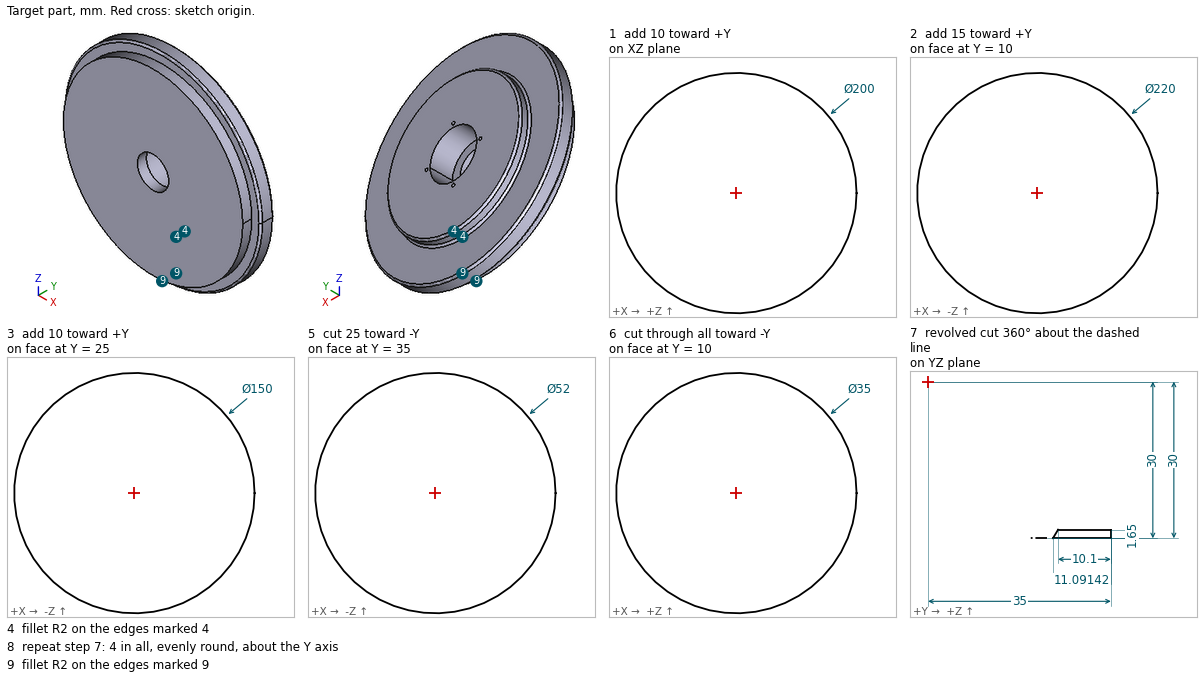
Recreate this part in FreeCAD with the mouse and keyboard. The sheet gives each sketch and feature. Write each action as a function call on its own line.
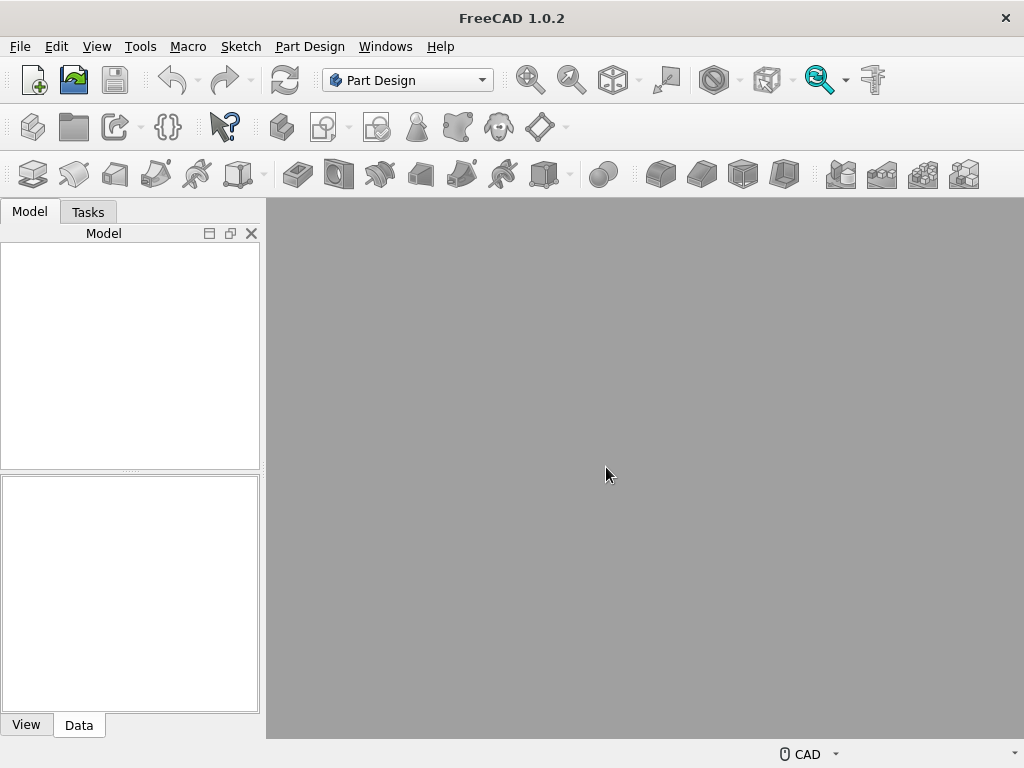
click(33, 80)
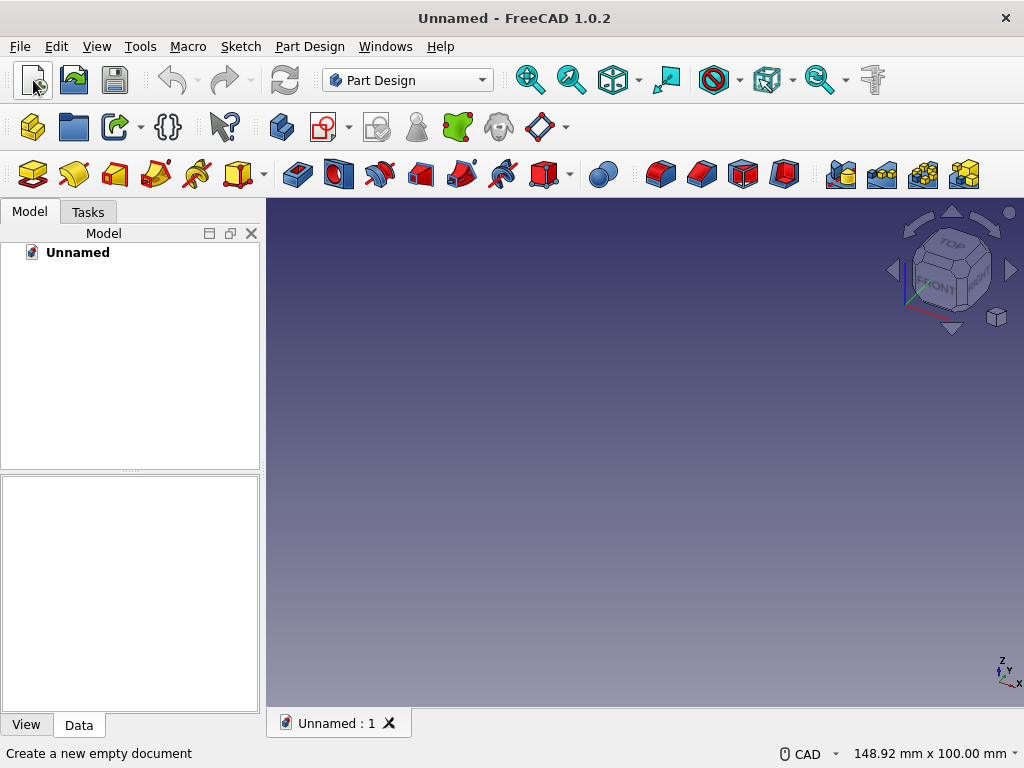
click(322, 128)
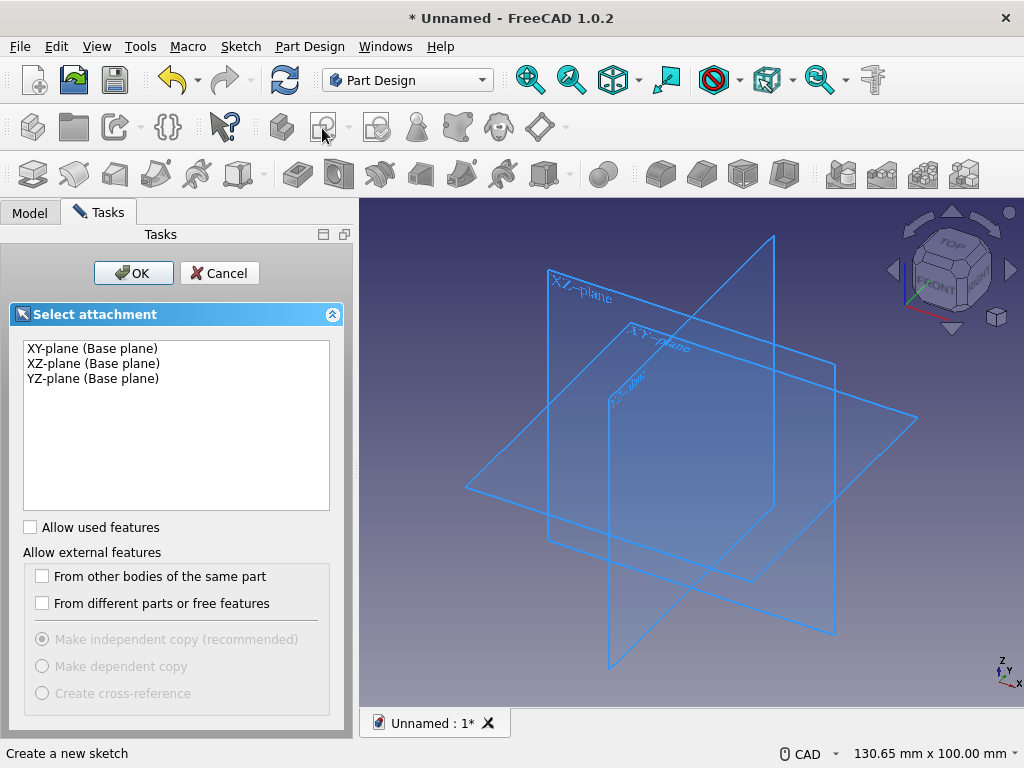
click(84, 364)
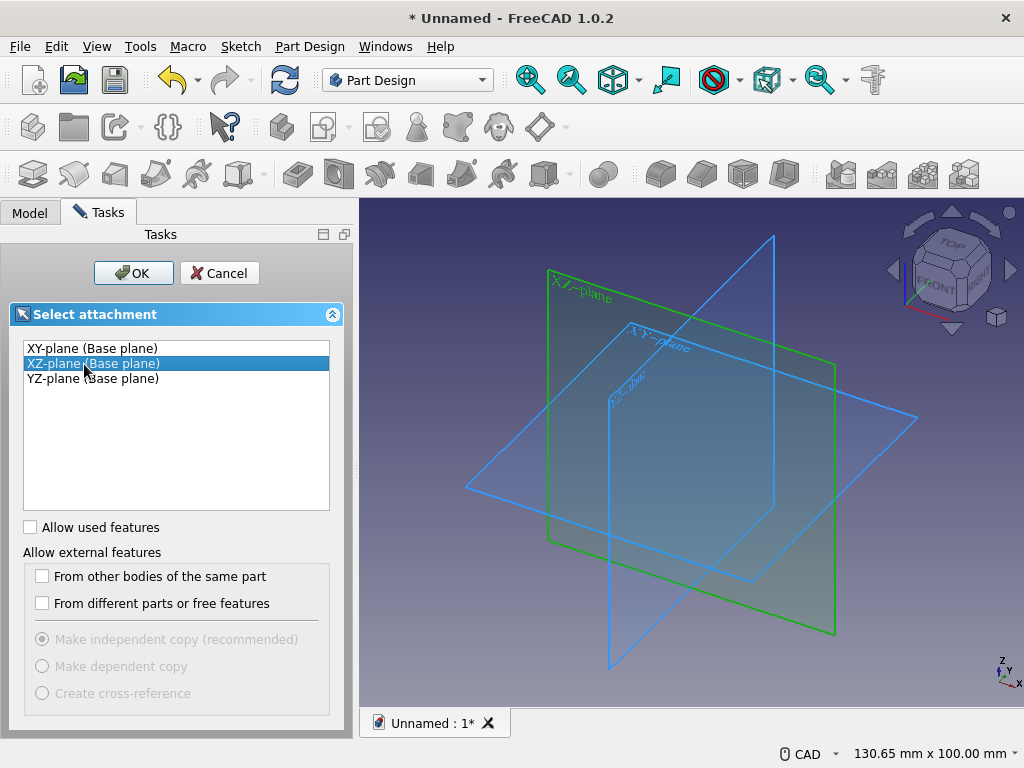
click(134, 273)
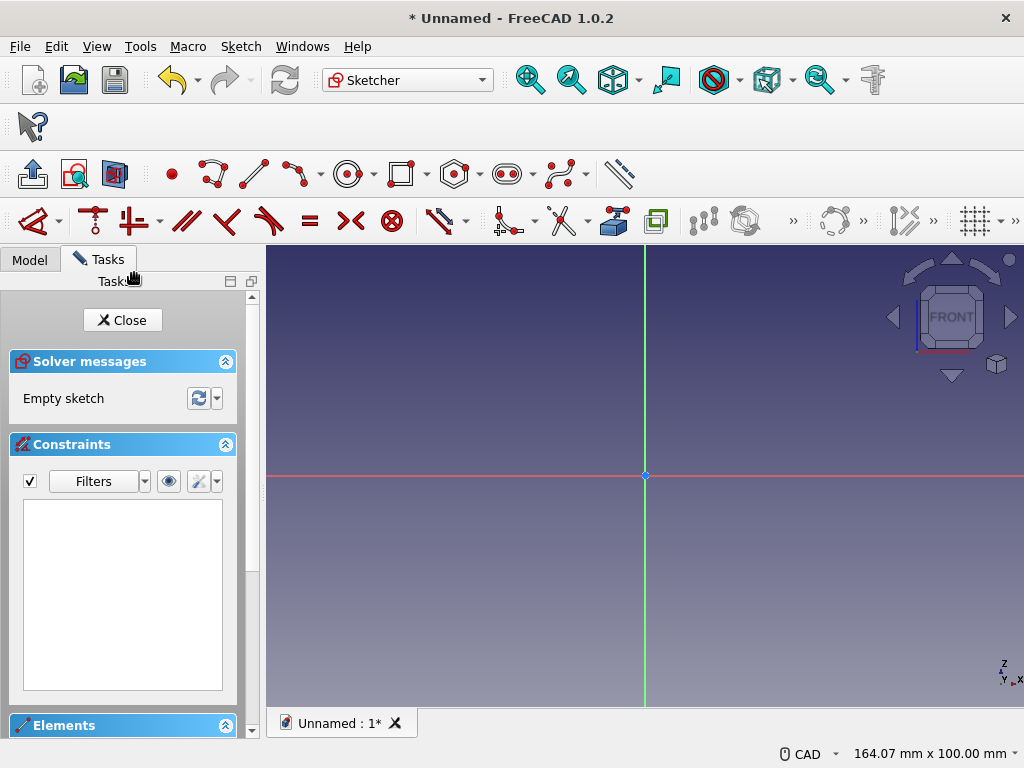
scroll(547, 476, down, 6)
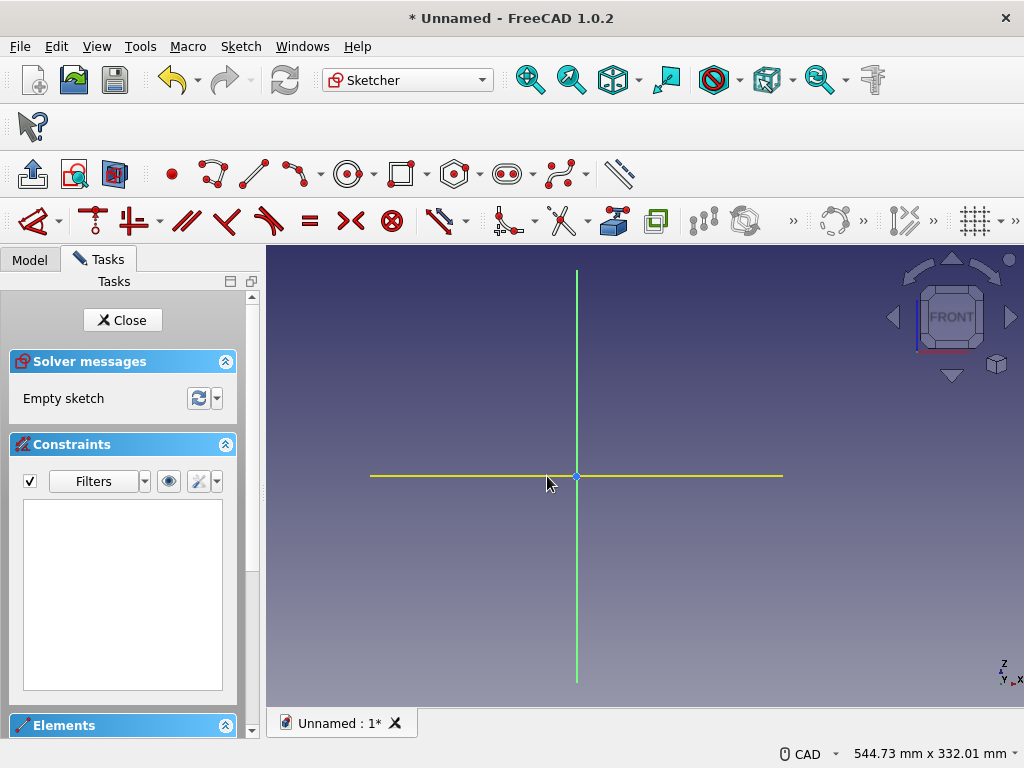
click(348, 174)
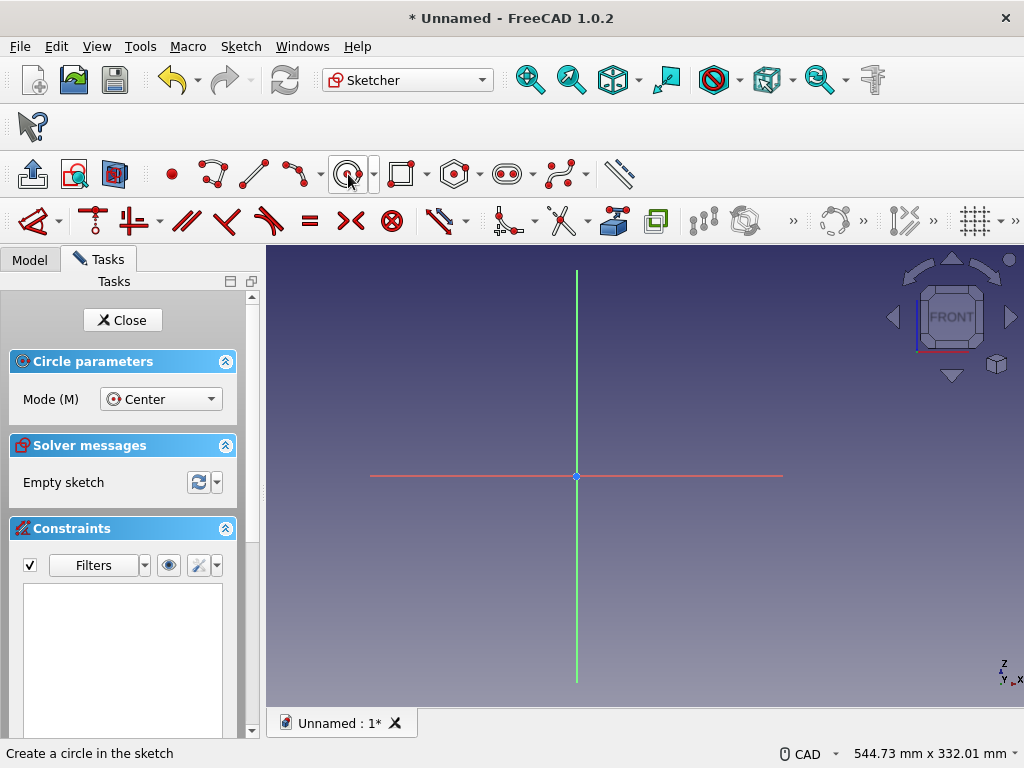
click(577, 476)
click(675, 378)
key(Escape)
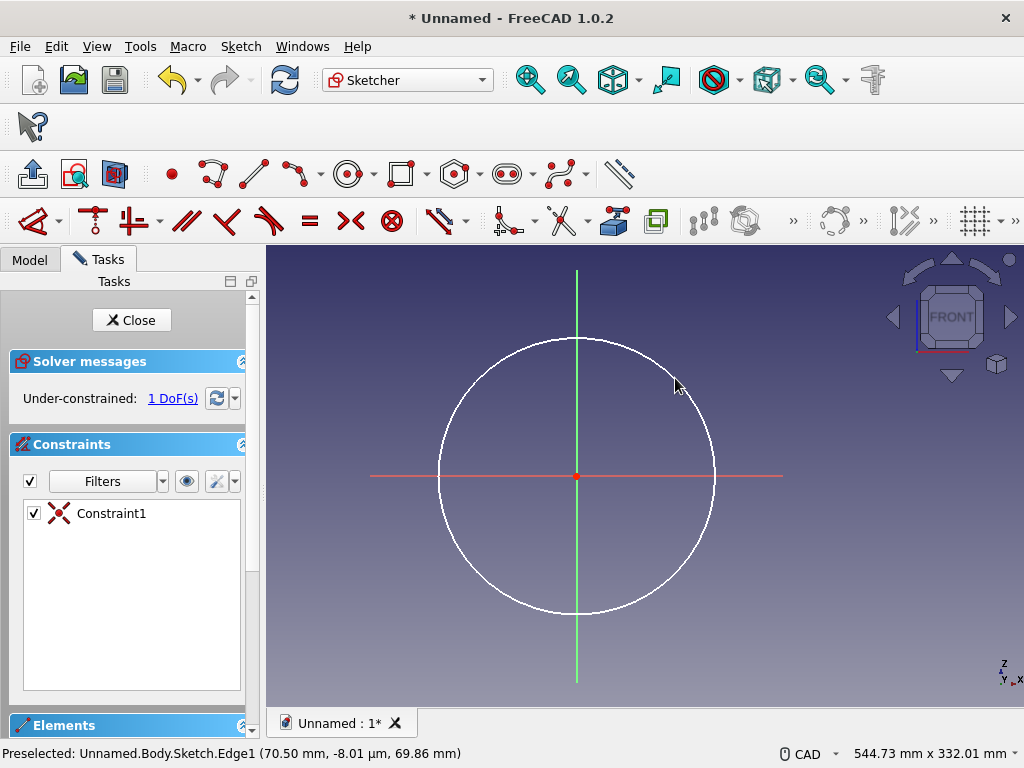
click(32, 222)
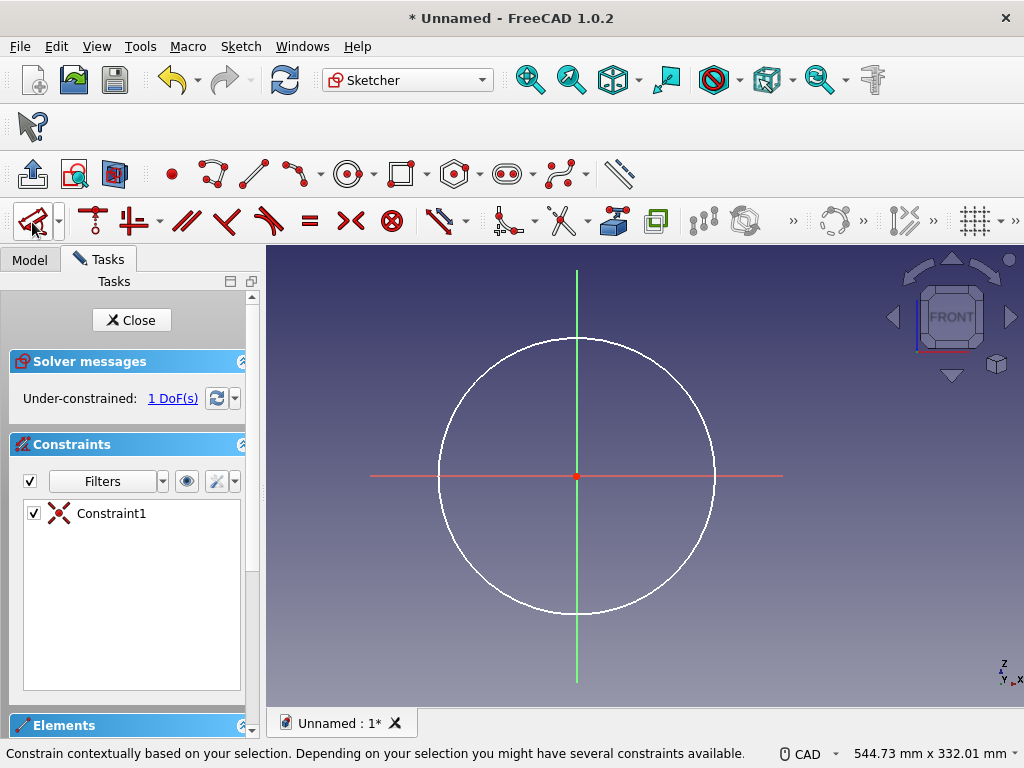
click(674, 378)
click(696, 355)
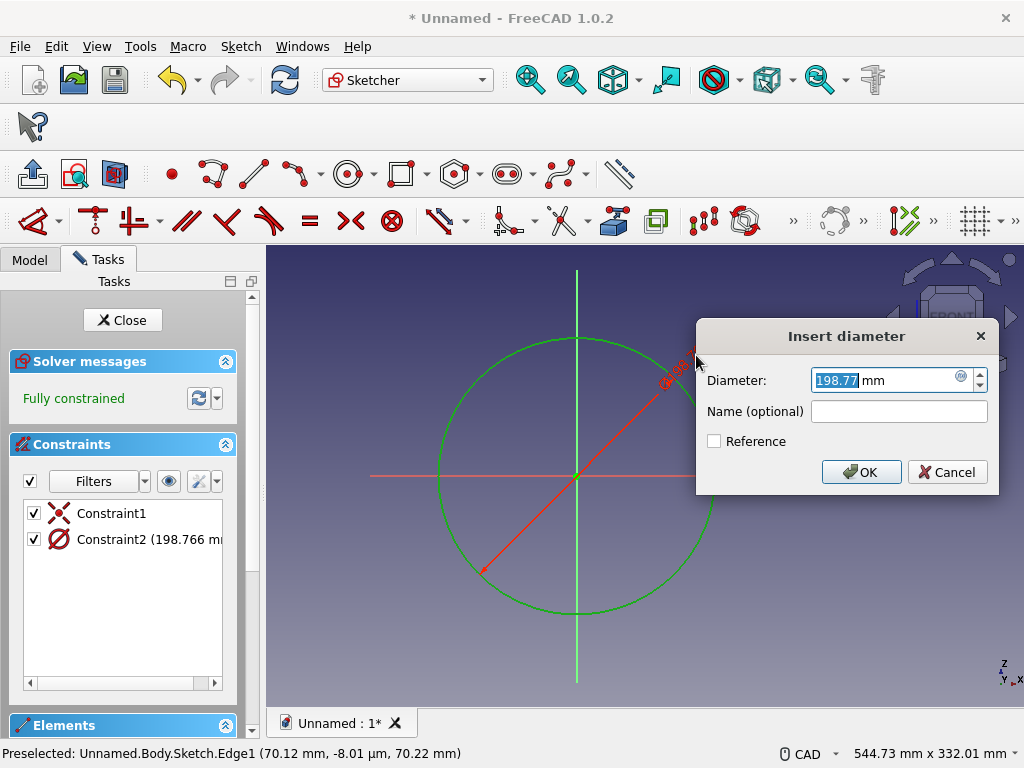
text(200)
key(Return)
key(Escape)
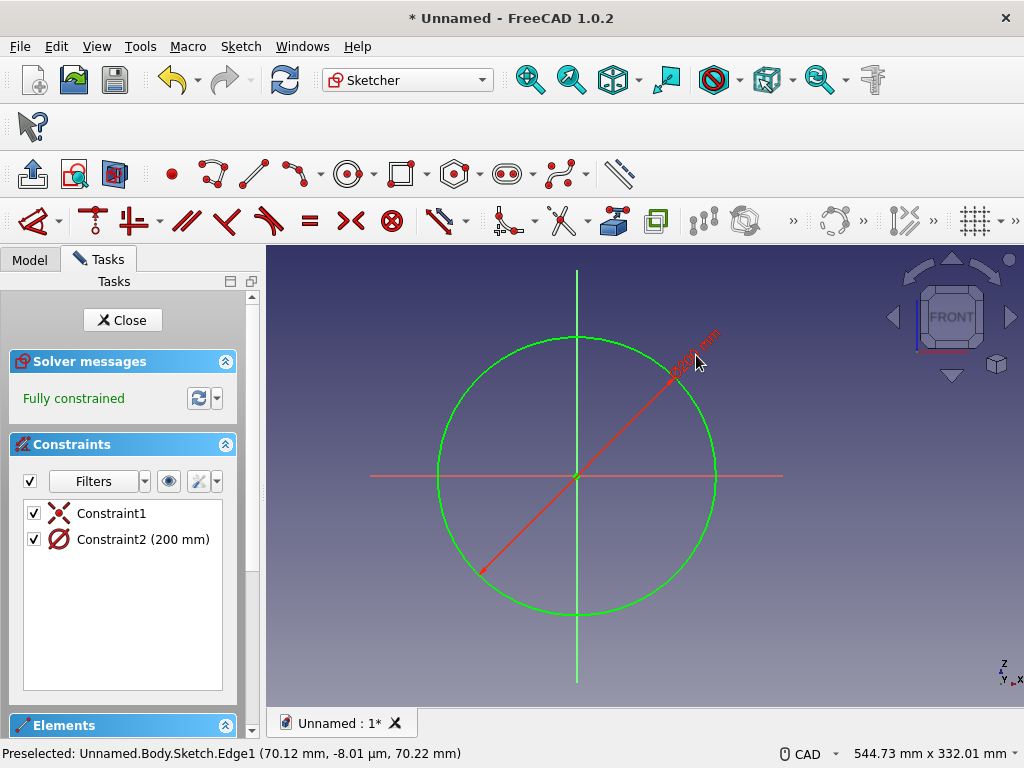
click(123, 320)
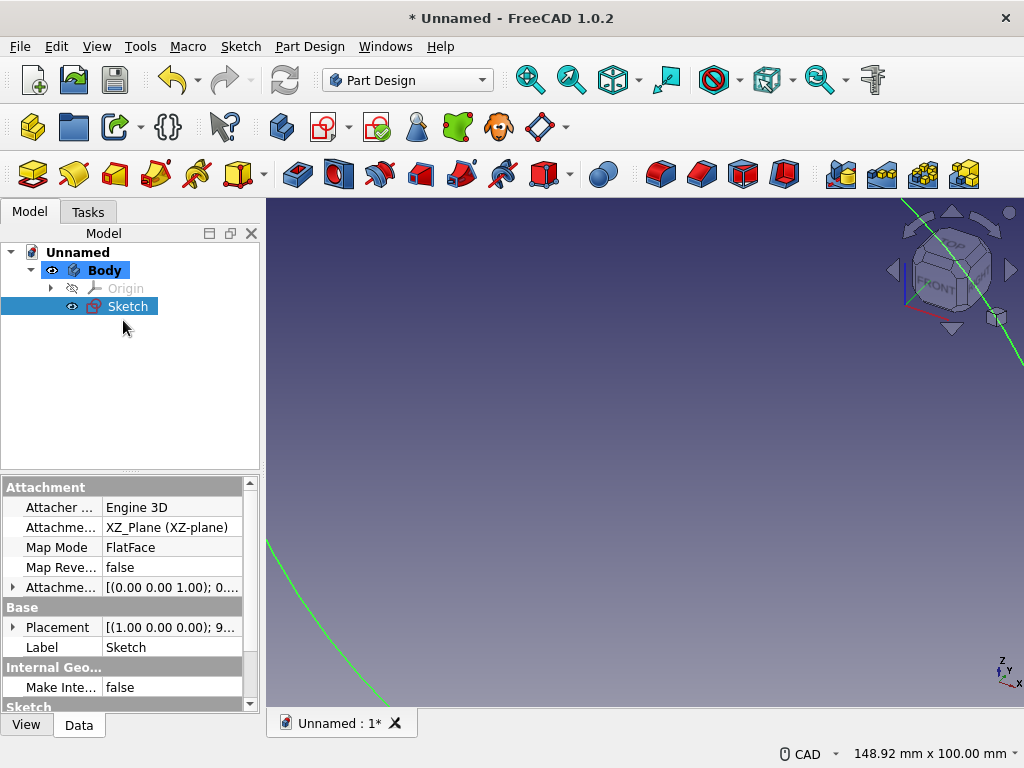
click(33, 174)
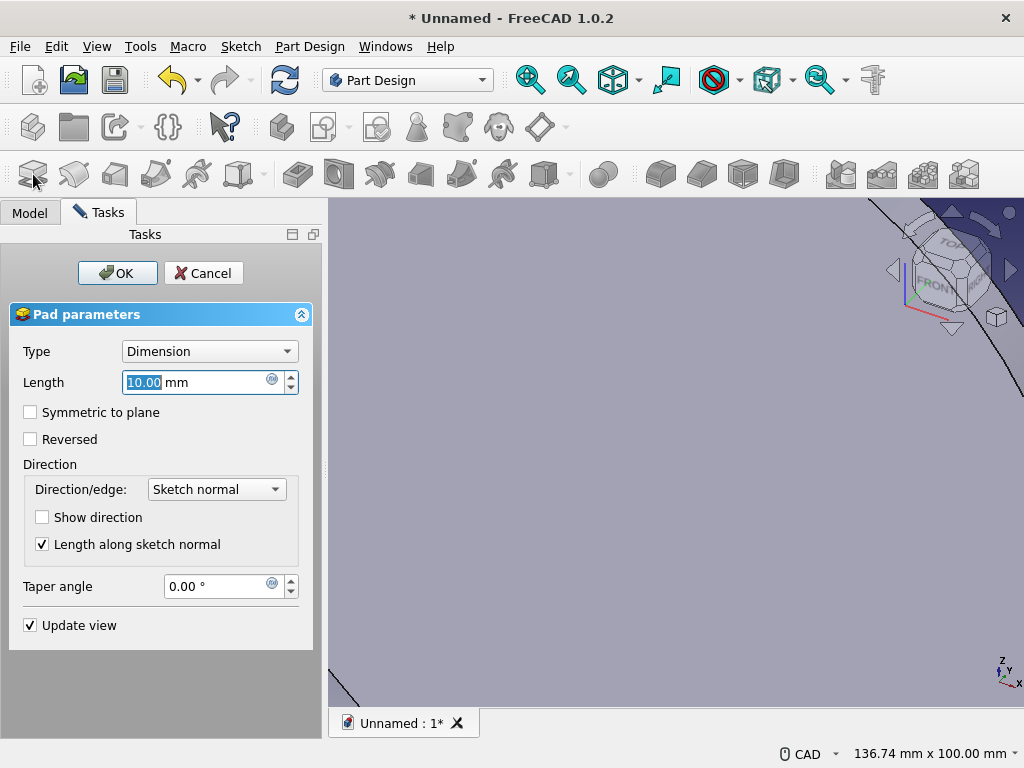
text(10)
key(Tab)